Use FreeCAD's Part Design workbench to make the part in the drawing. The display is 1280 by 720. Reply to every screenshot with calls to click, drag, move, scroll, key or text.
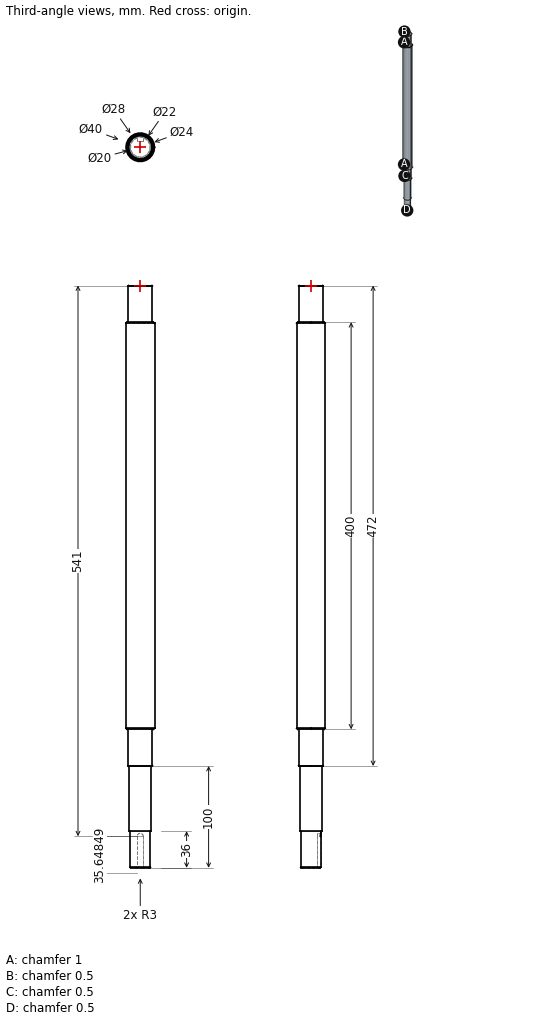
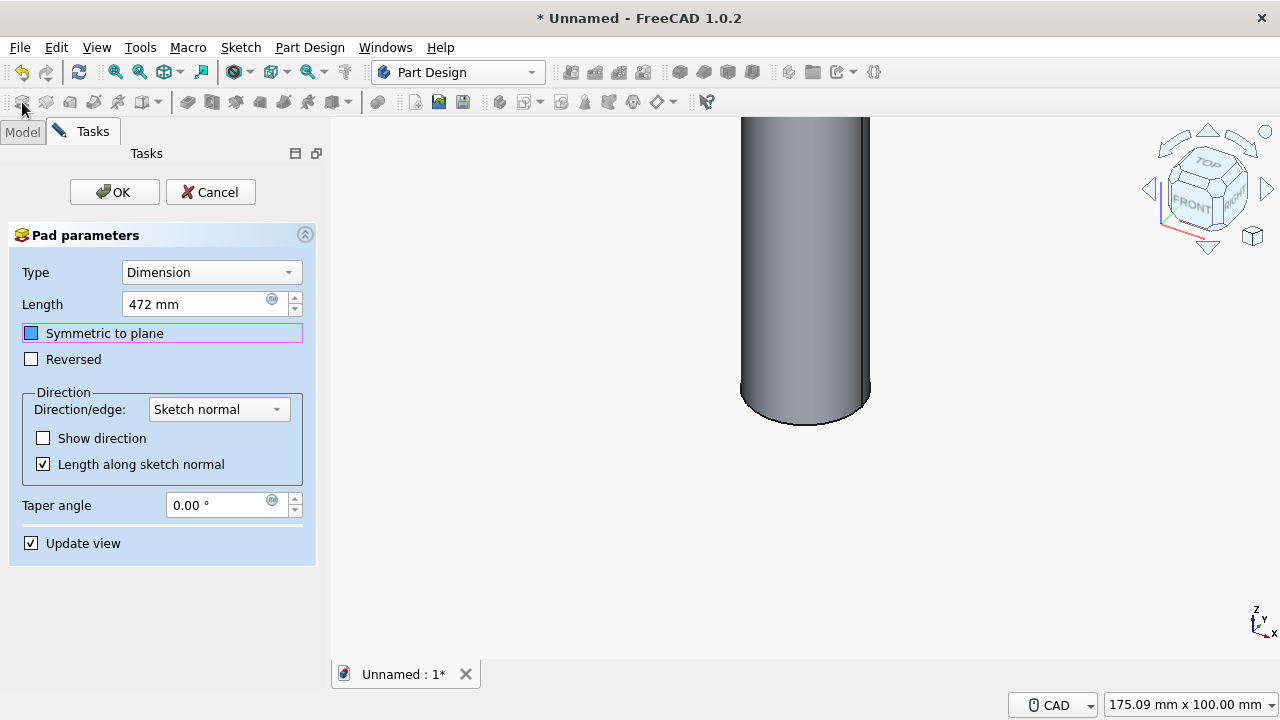
click(30, 359)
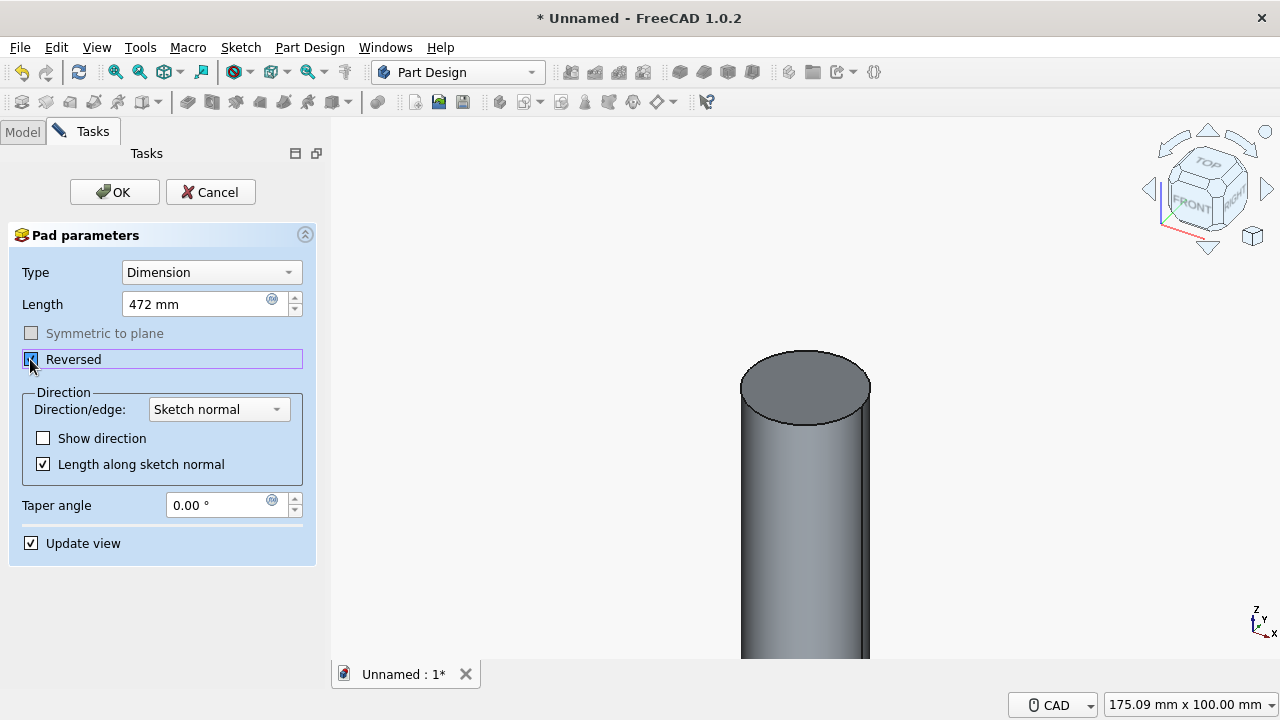
click(115, 192)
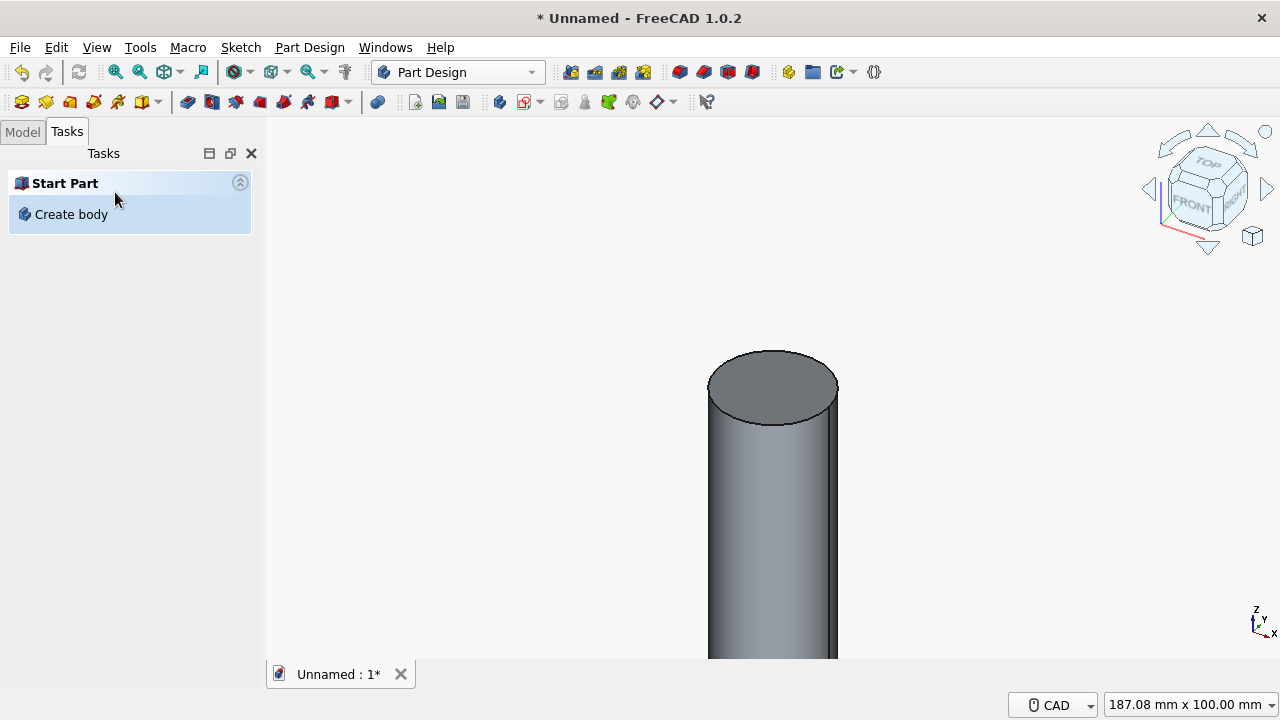
click(116, 72)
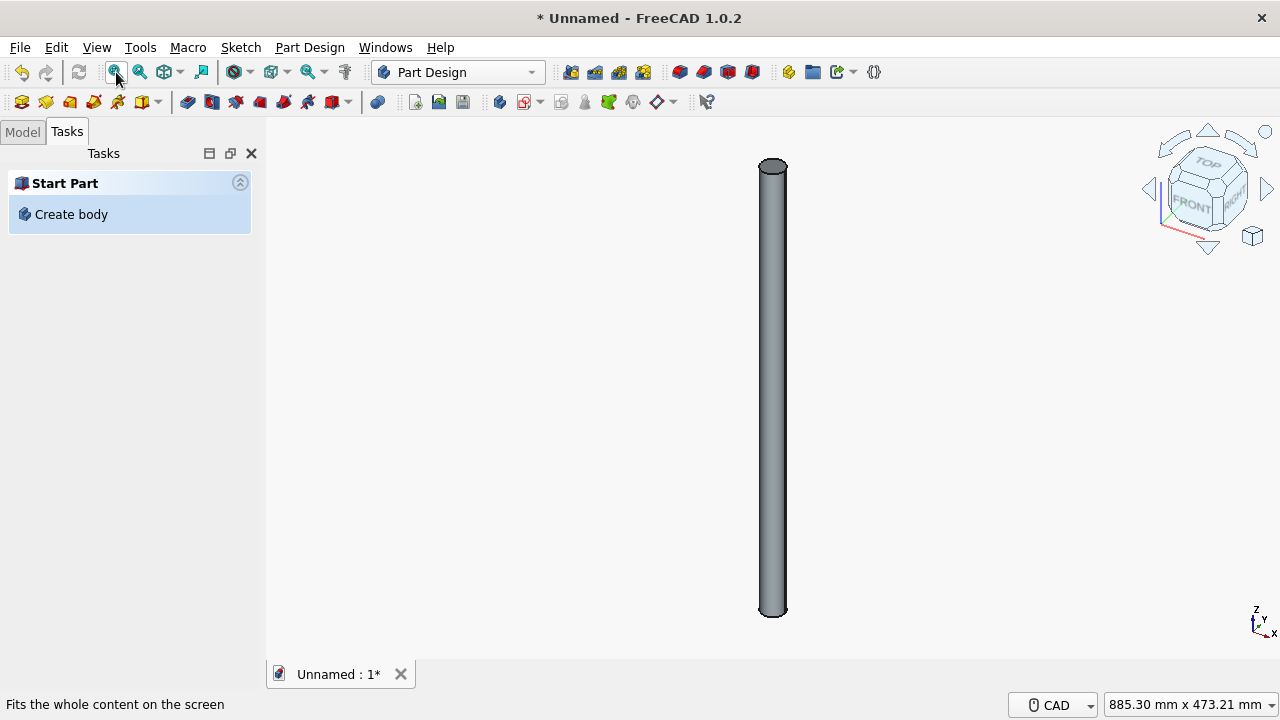
key(5)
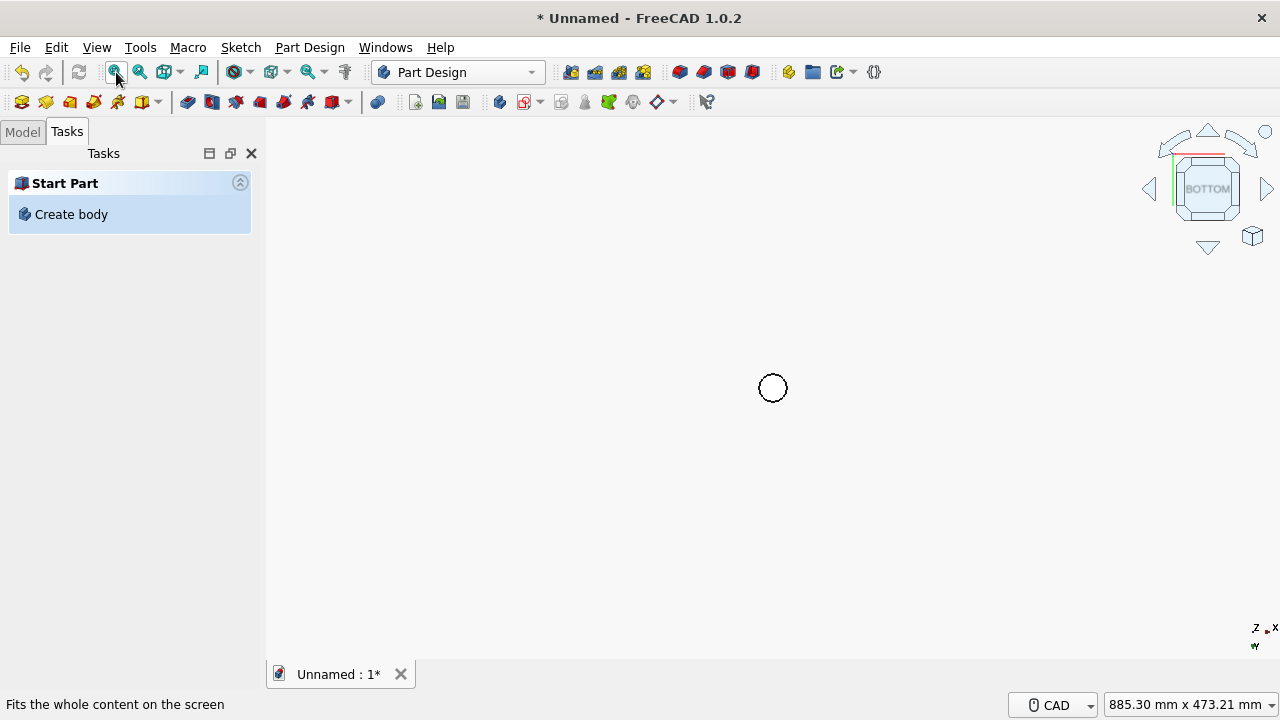
click(116, 72)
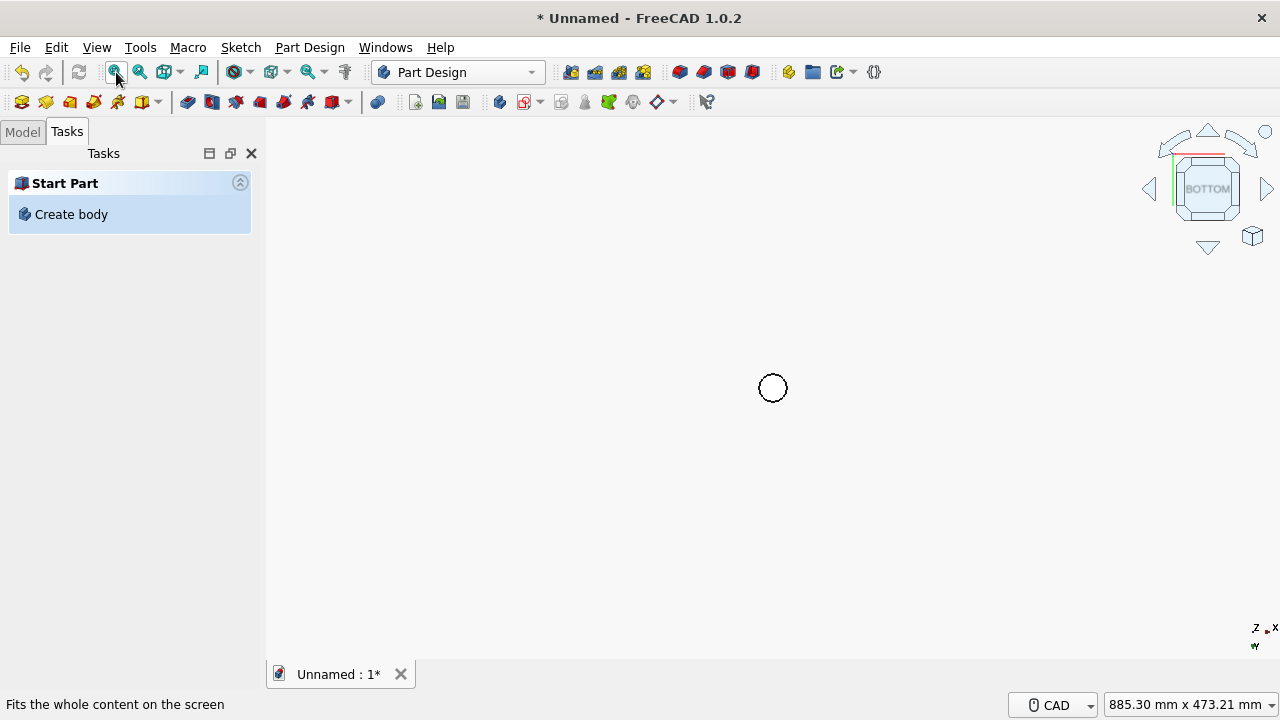
click(773, 387)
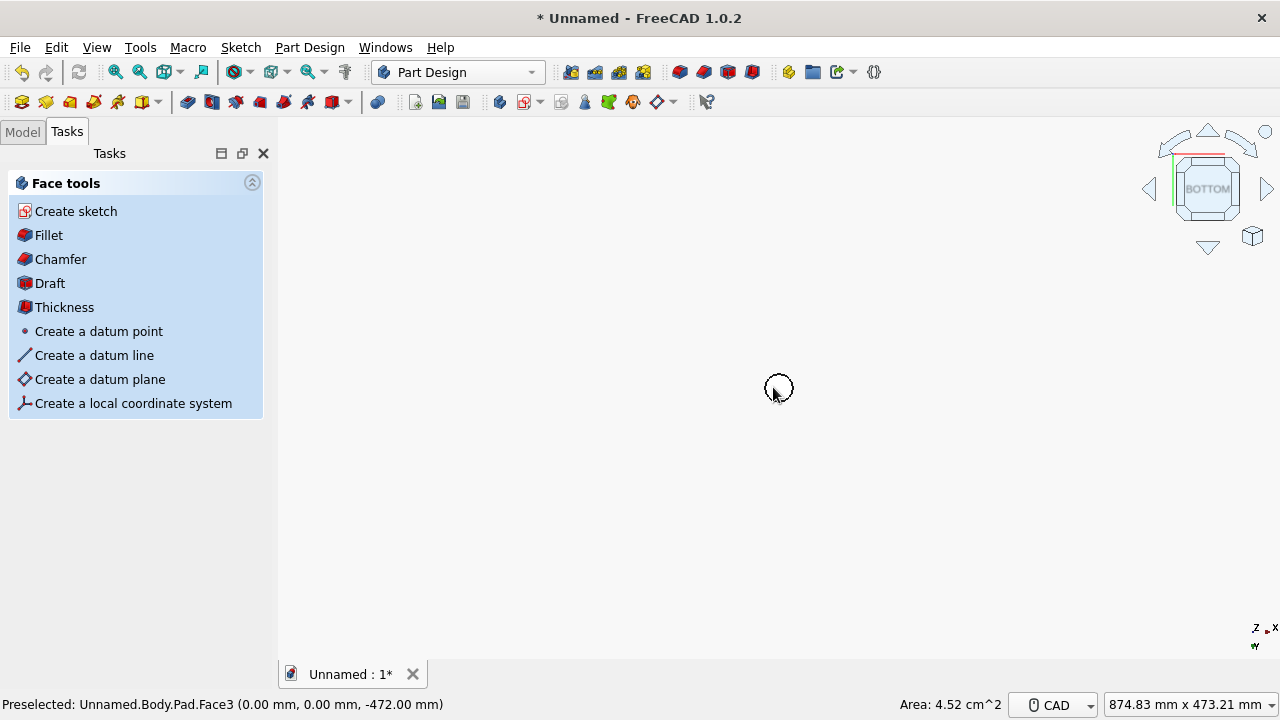
click(524, 102)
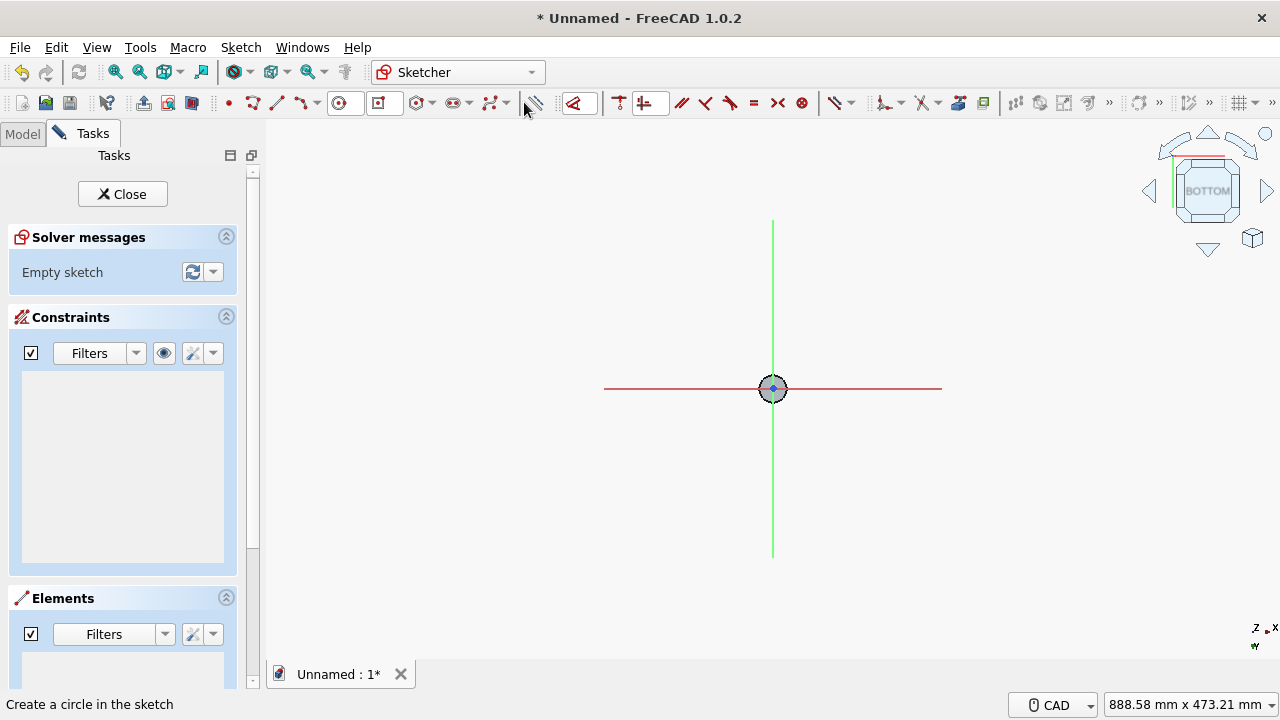
scroll(778, 389, up, 13)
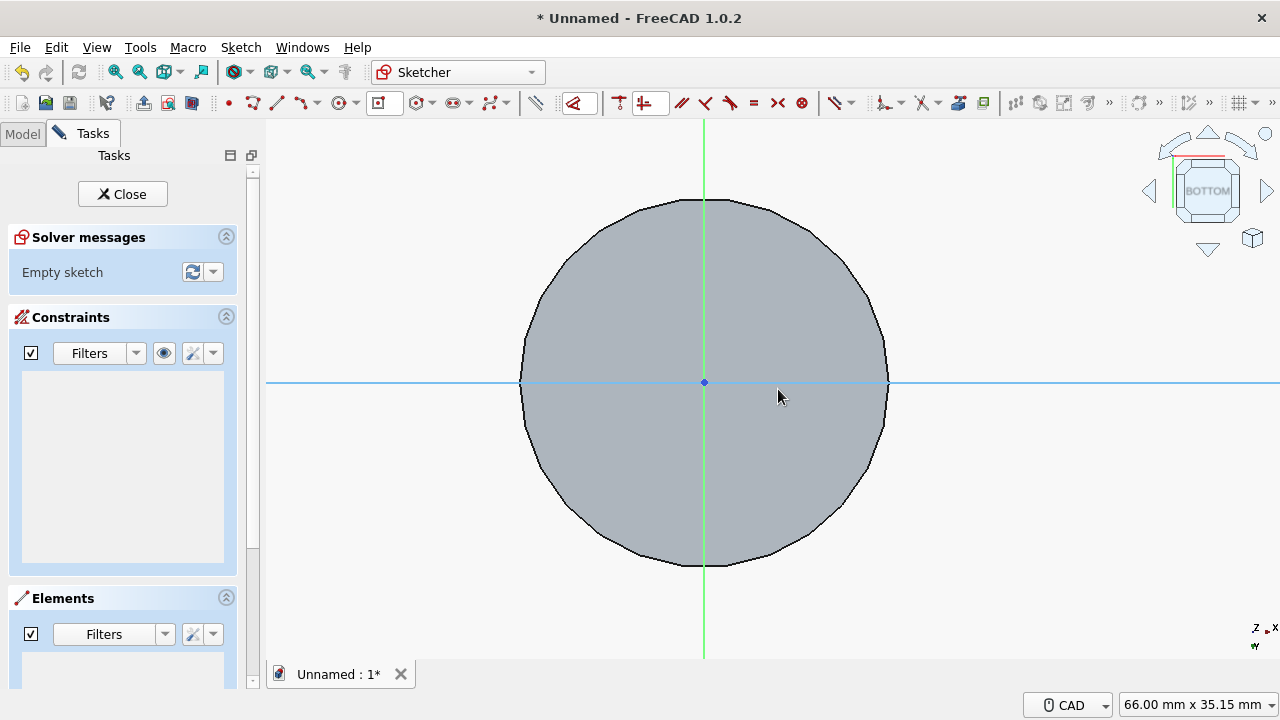
click(340, 104)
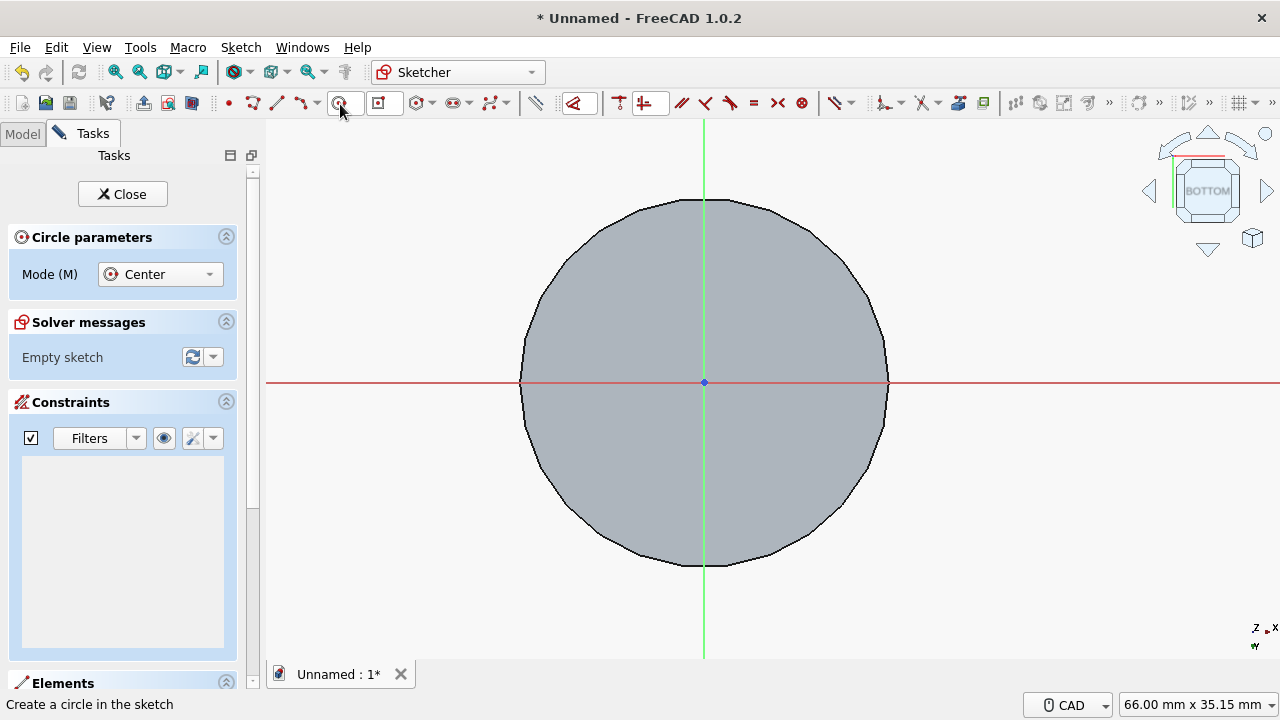
click(704, 383)
move(824, 263)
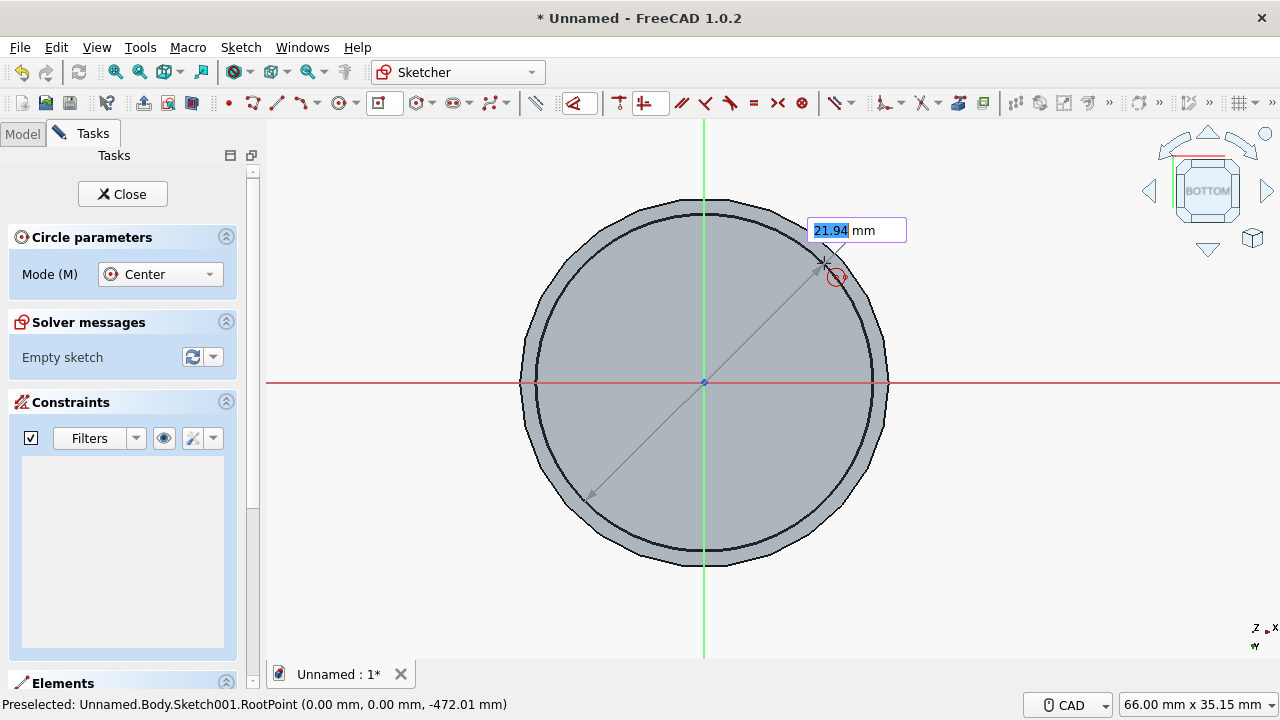
text(22)
key(Return)
key(Escape)